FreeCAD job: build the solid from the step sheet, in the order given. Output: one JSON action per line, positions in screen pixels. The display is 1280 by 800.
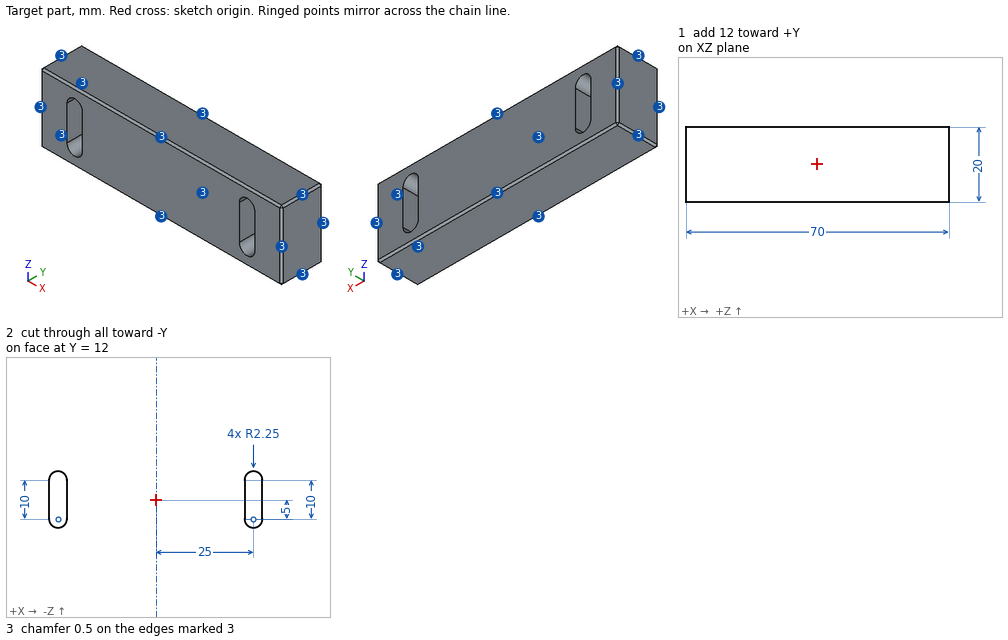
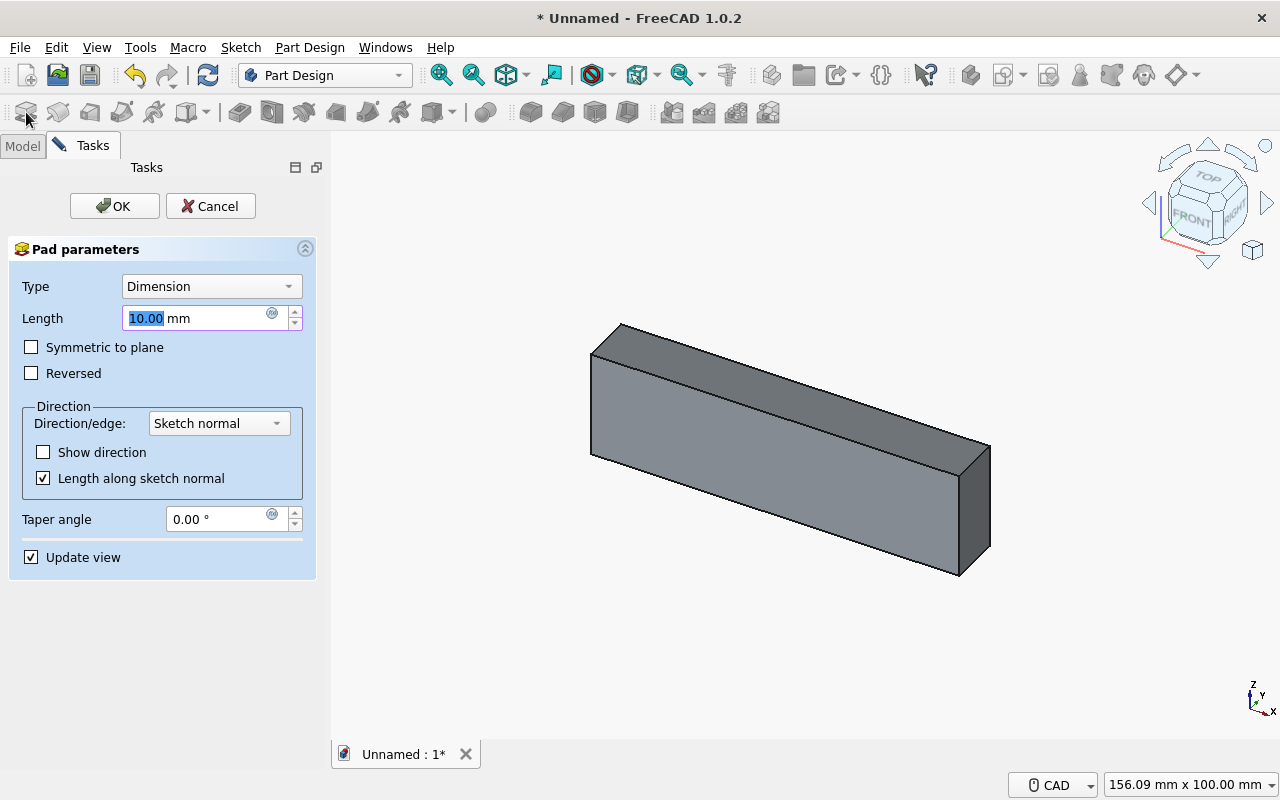
{"action": "type", "text": "12"}
{"action": "key", "text": "Tab"}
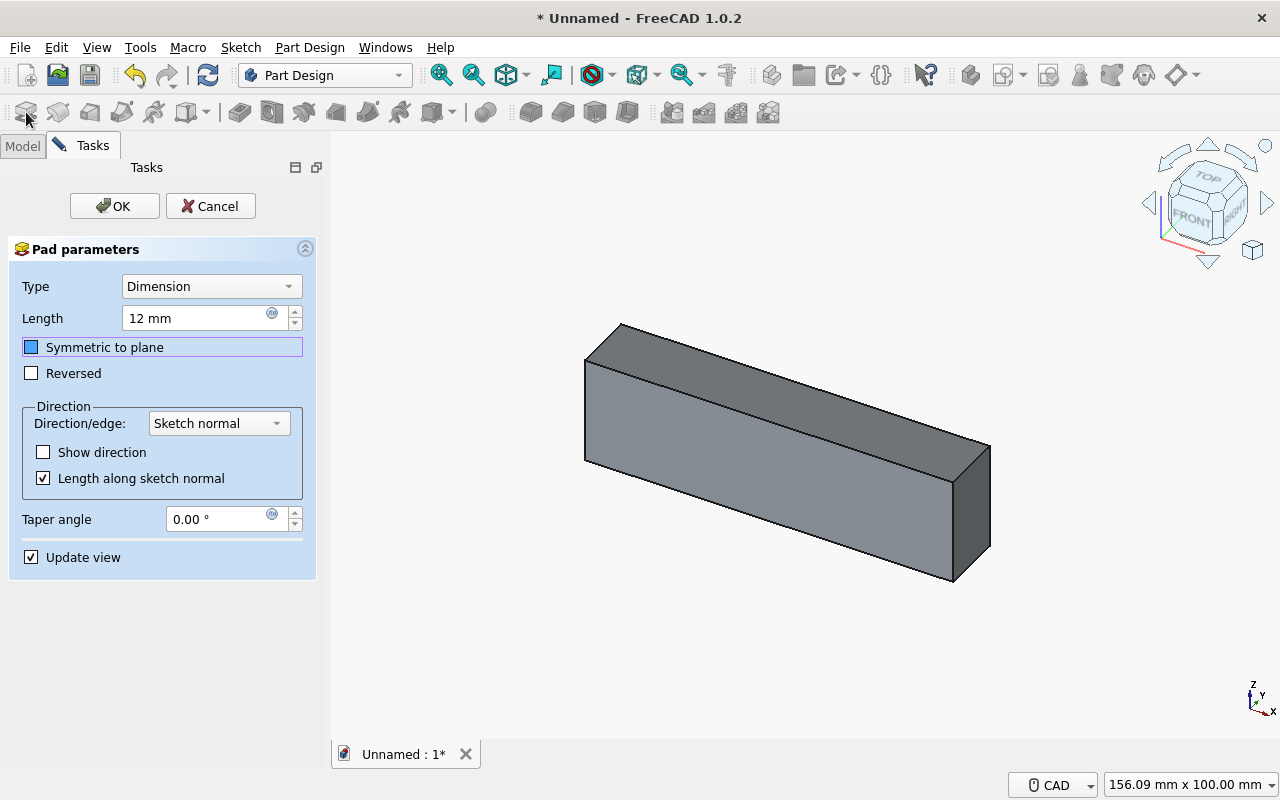
{"action": "left_click", "coordinate": [30, 373]}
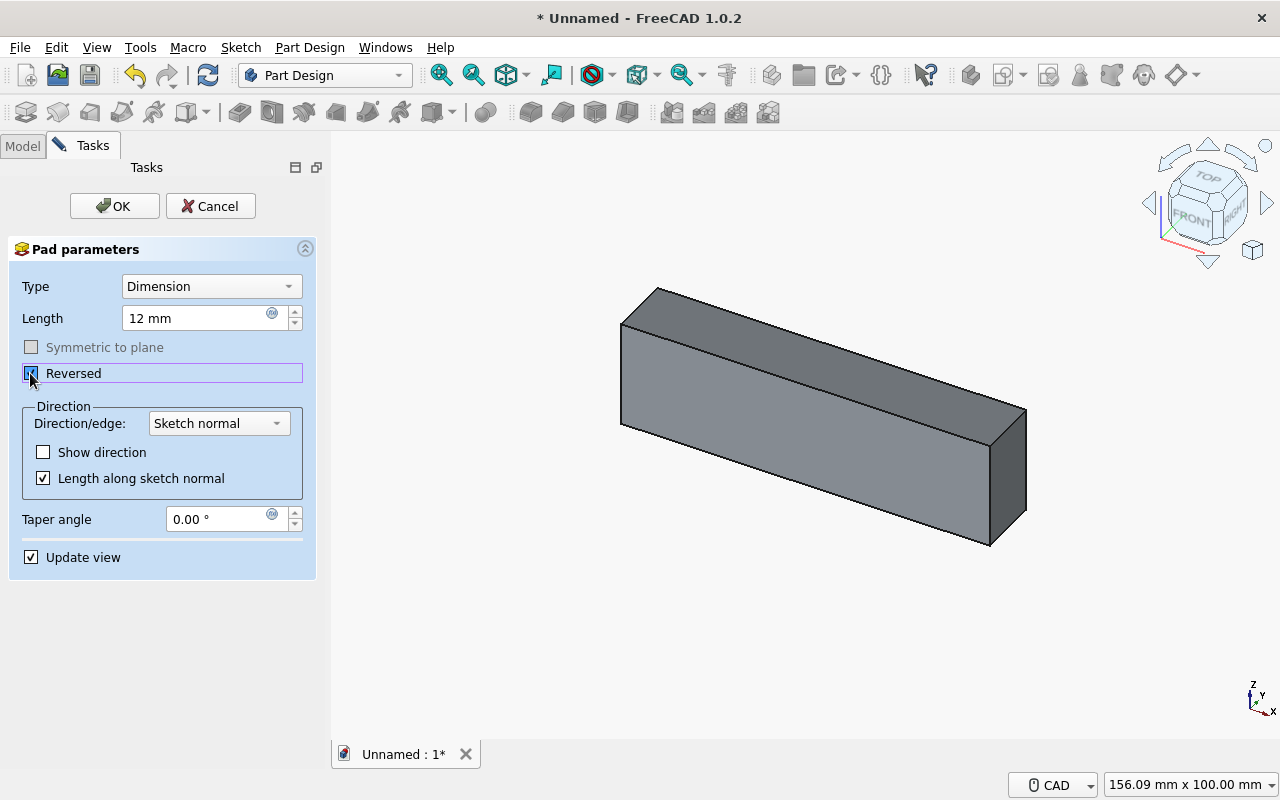
{"action": "left_click", "coordinate": [115, 206]}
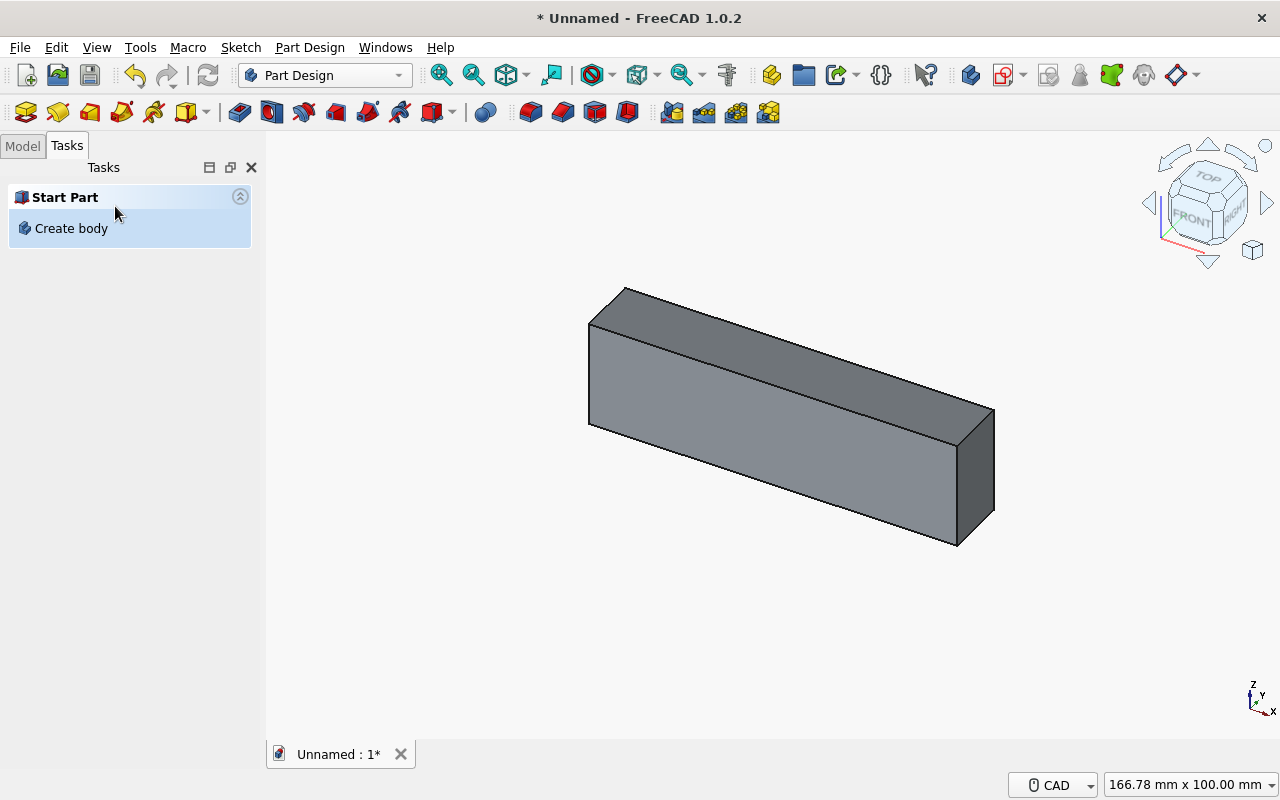
{"action": "key", "text": "v f"}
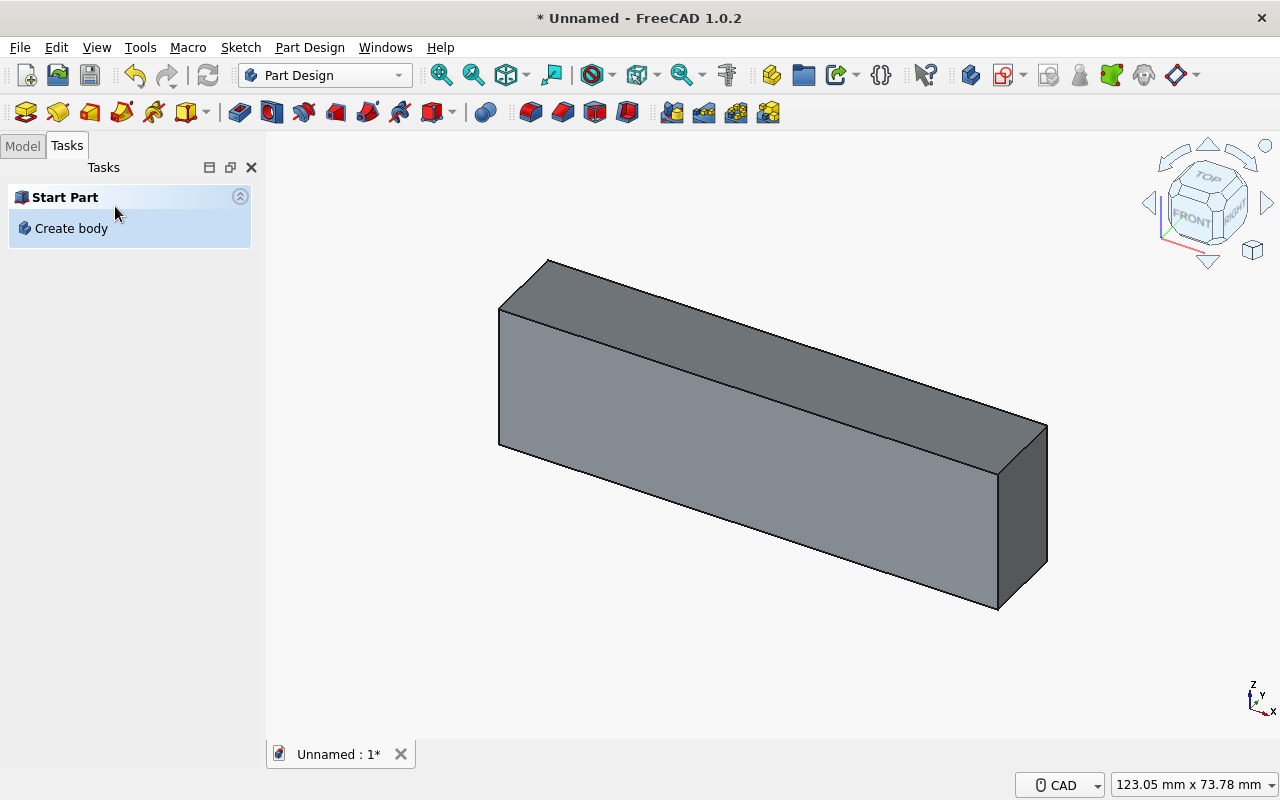
{"action": "key", "text": "4"}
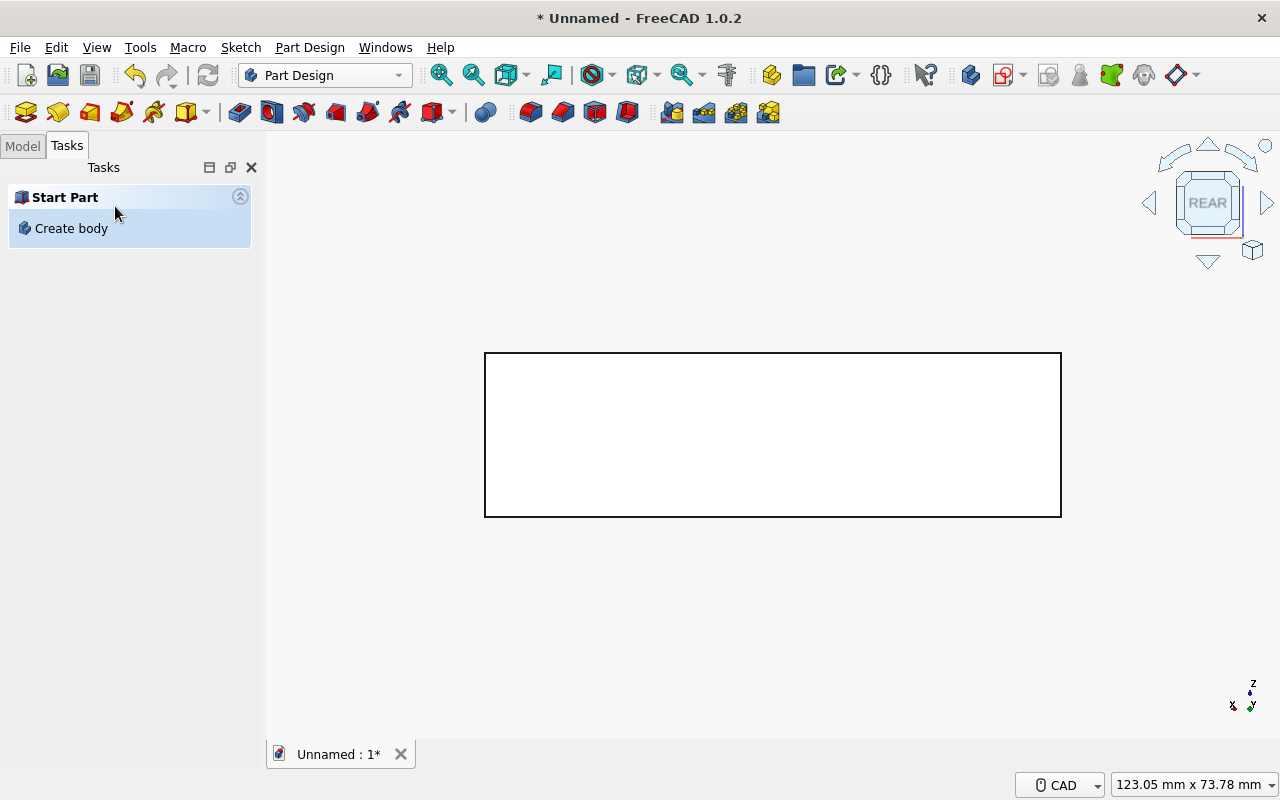
{"action": "left_click", "coordinate": [608, 434]}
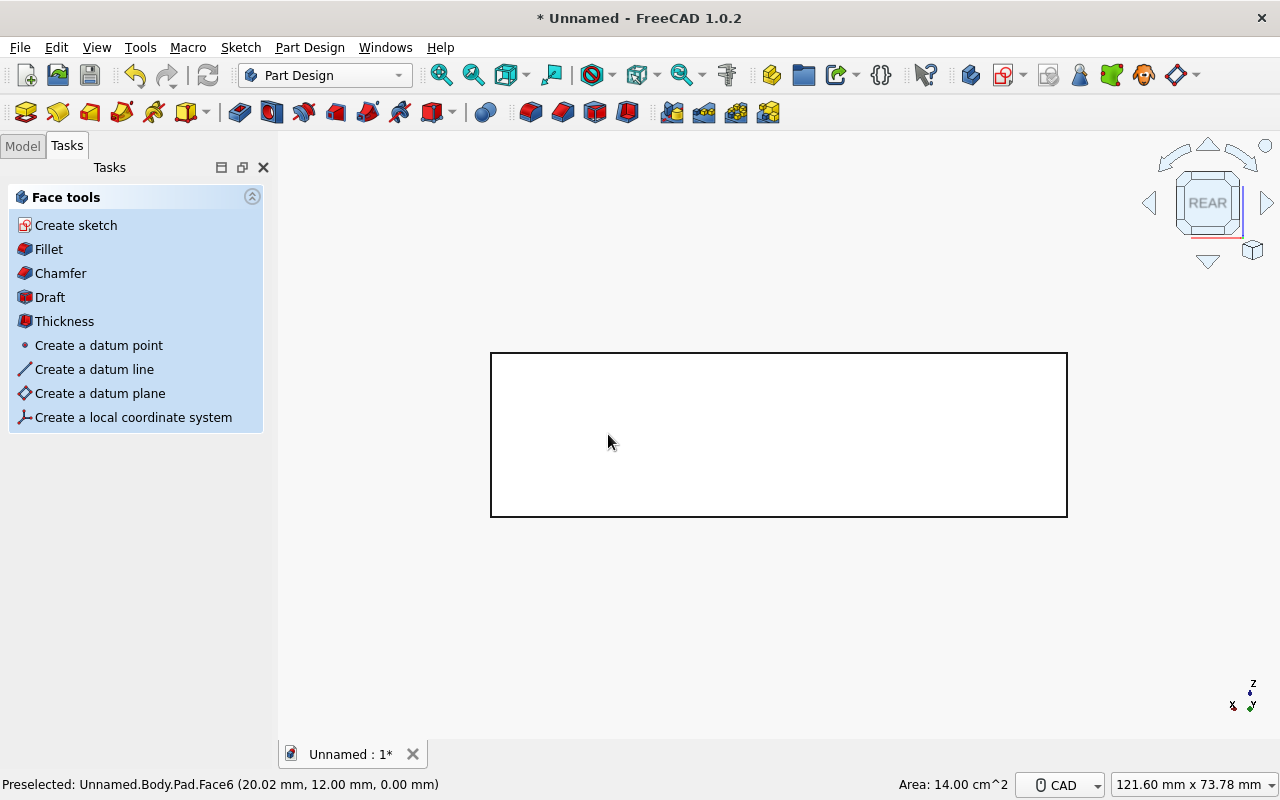
{"action": "left_click", "coordinate": [1004, 76]}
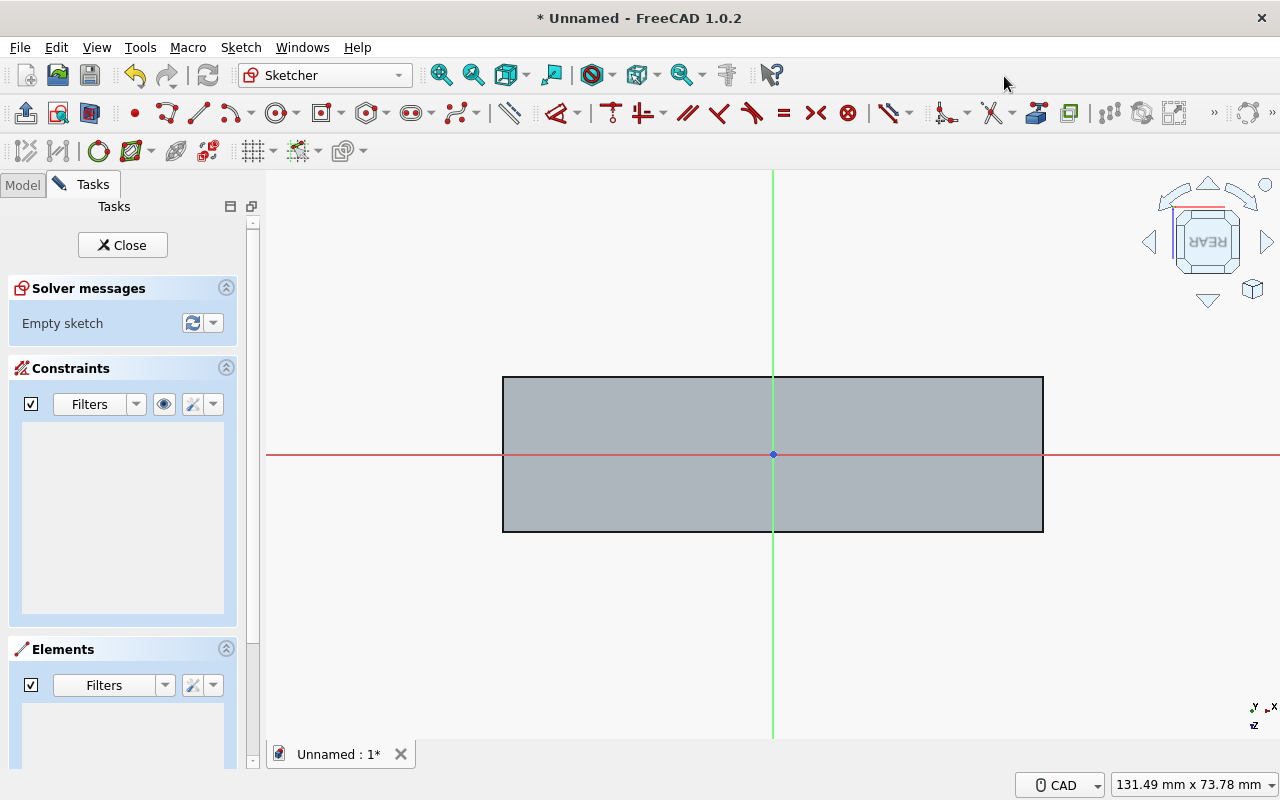
{"action": "scroll", "coordinate": [912, 455], "scroll_direction": "up", "scroll_amount": 2}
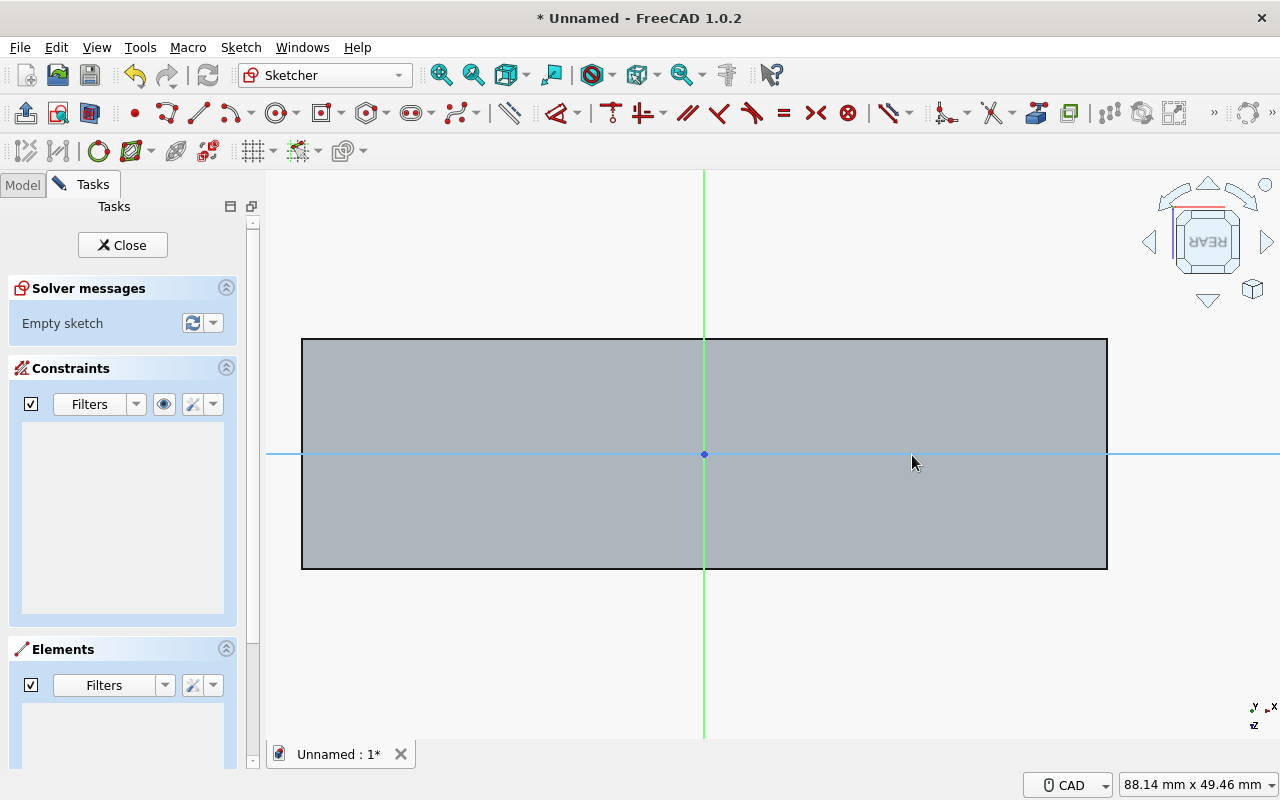
{"action": "key", "text": "g s"}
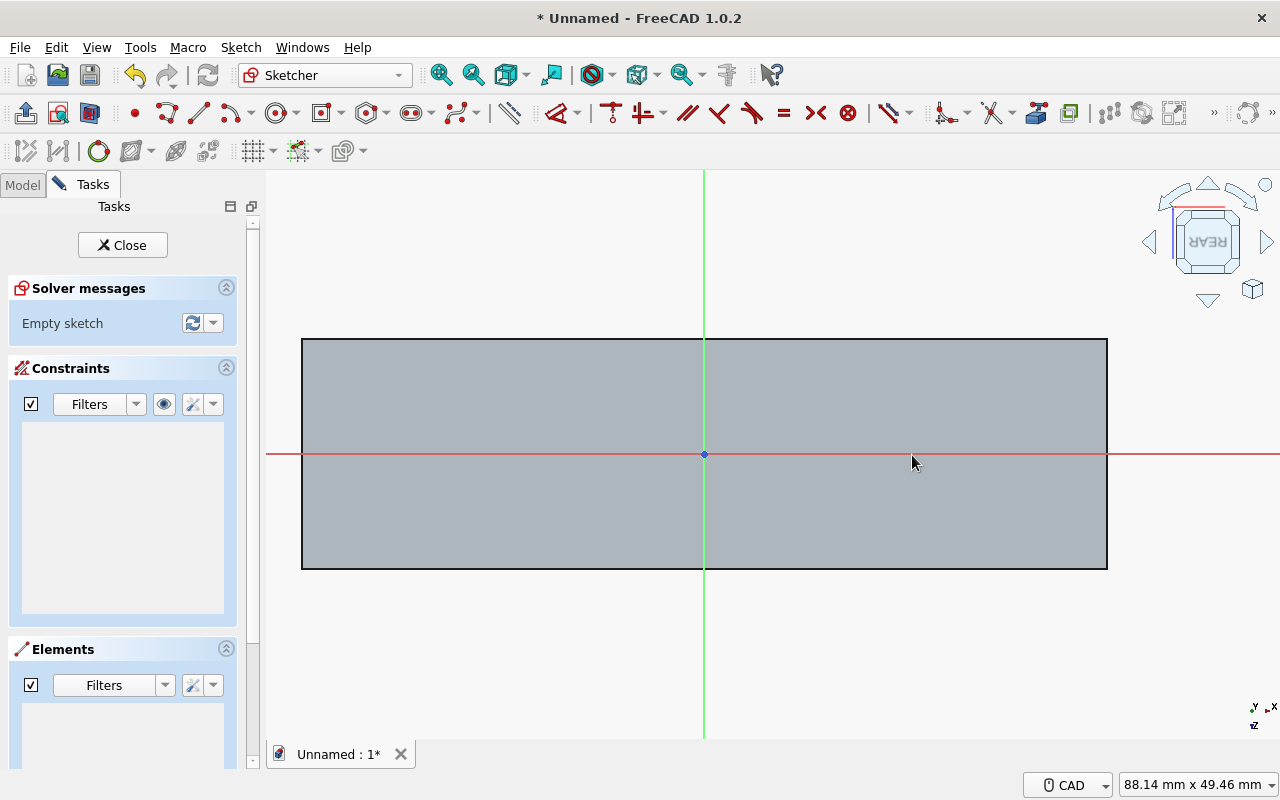
{"action": "left_click", "coordinate": [992, 512]}